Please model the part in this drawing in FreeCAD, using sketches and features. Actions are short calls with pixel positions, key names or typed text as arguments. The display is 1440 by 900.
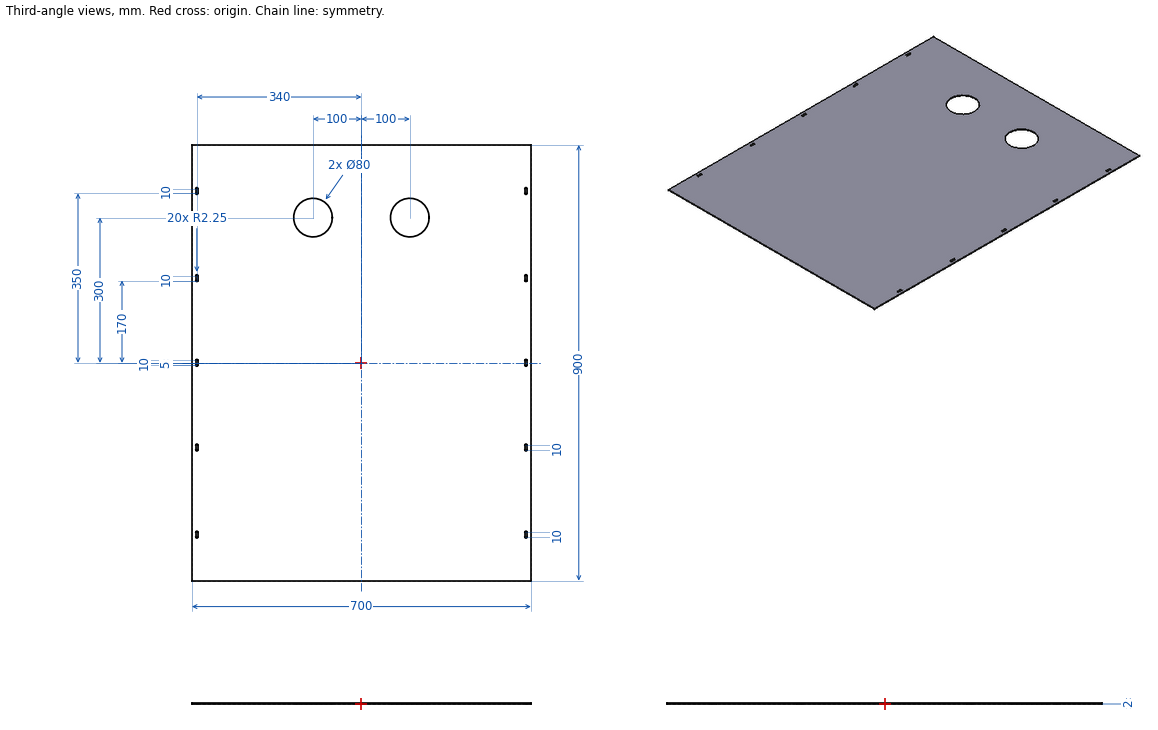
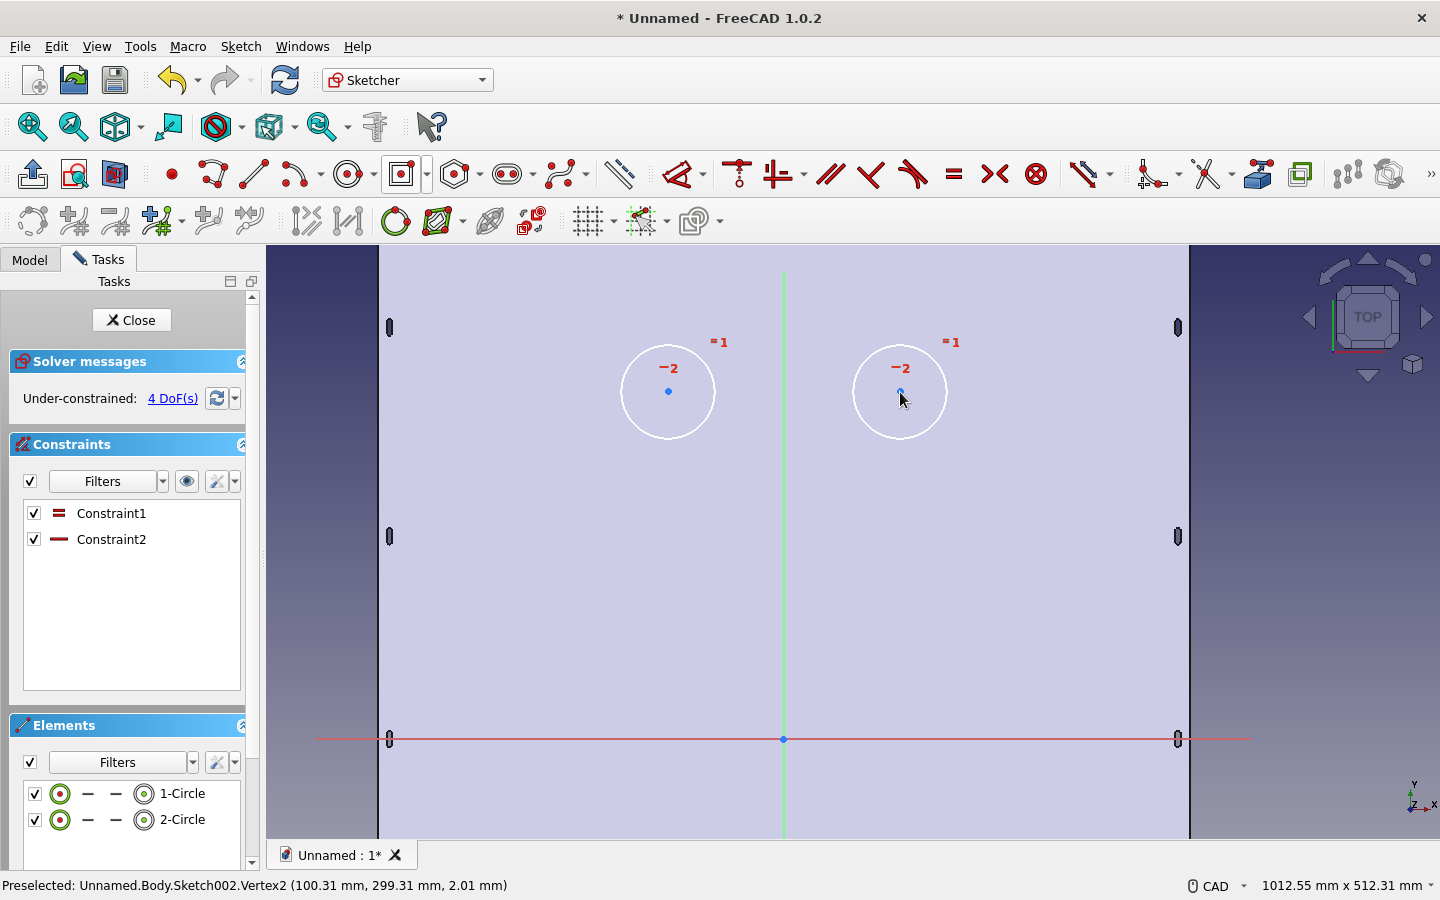
key(d)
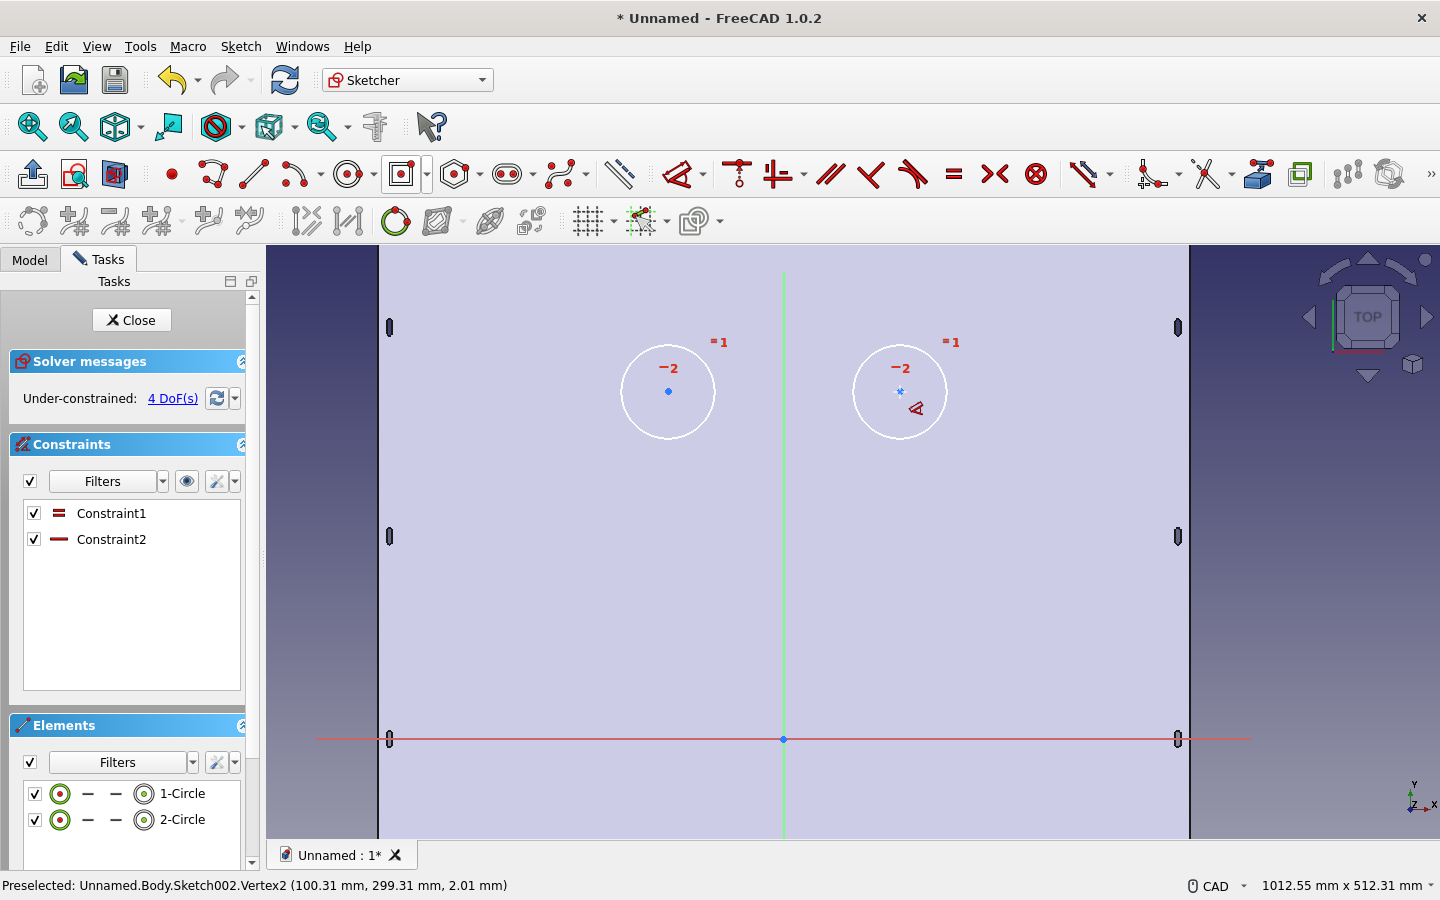
click(701, 359)
click(724, 336)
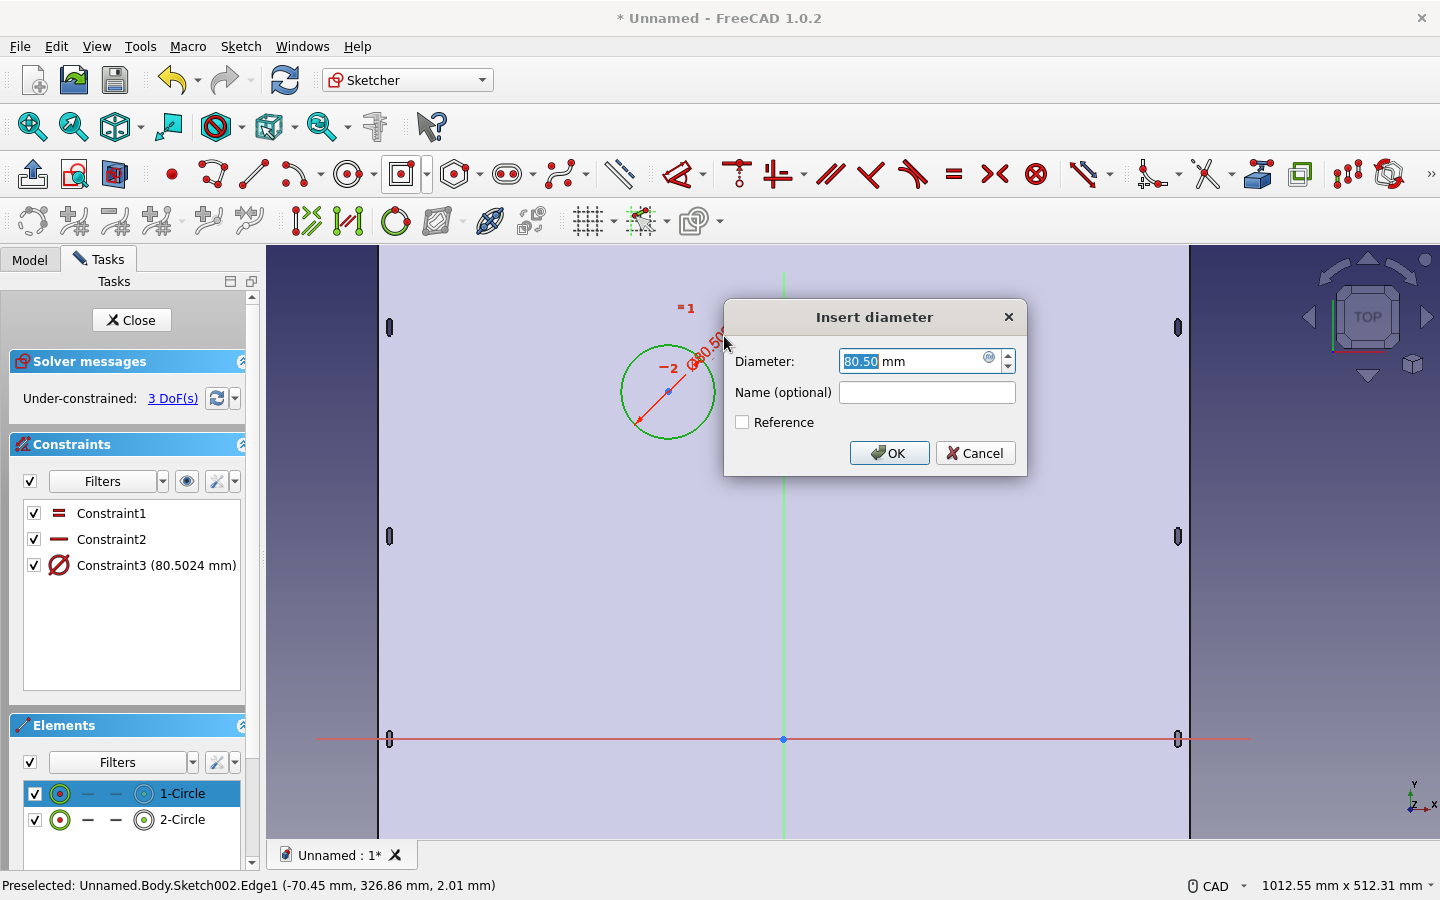
text(80)
key(Return)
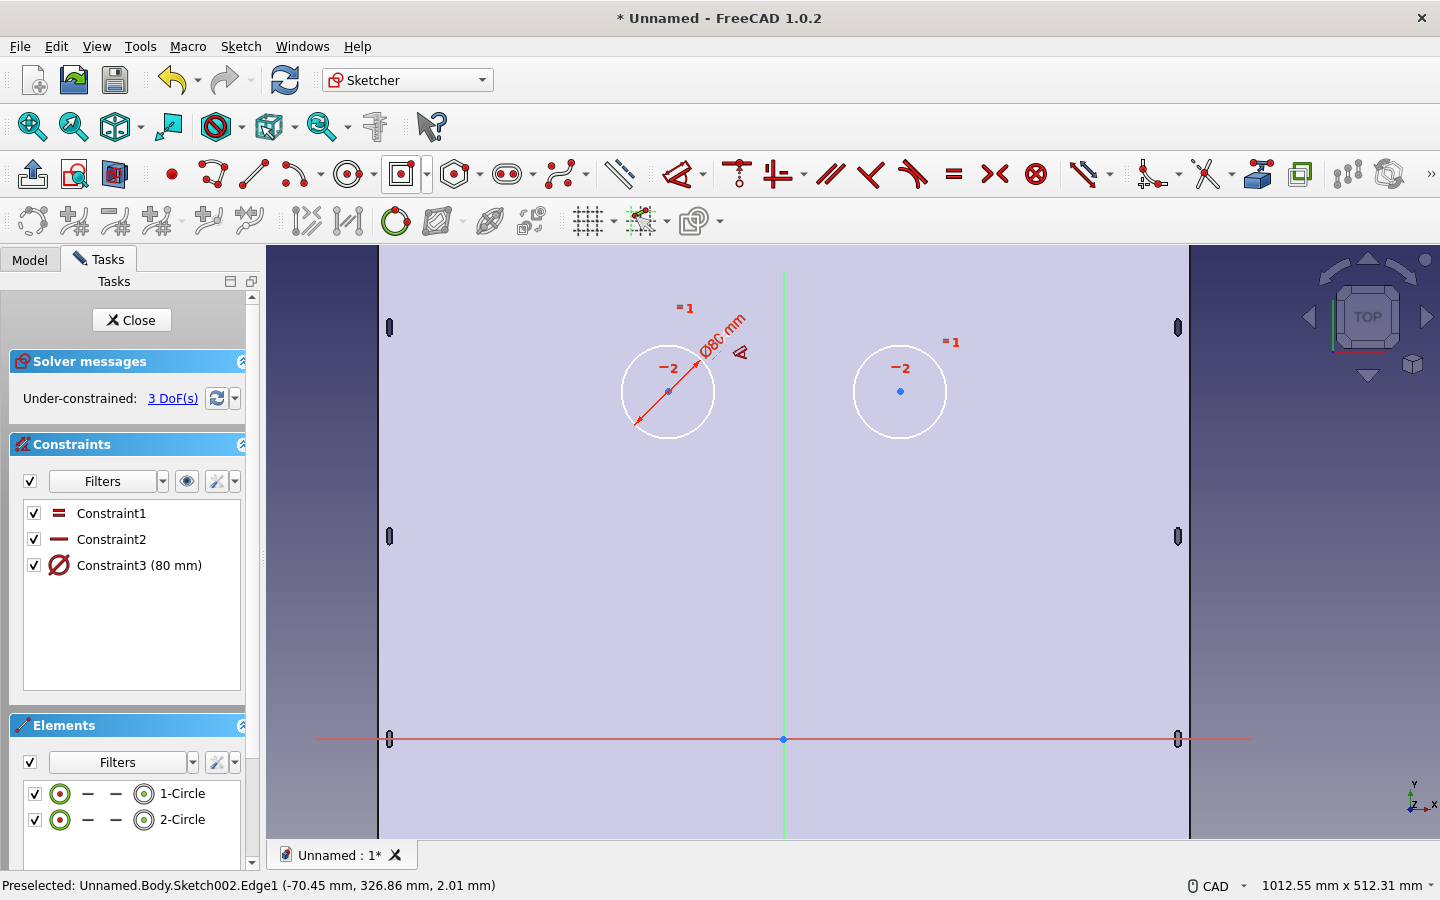
click(668, 392)
click(726, 773)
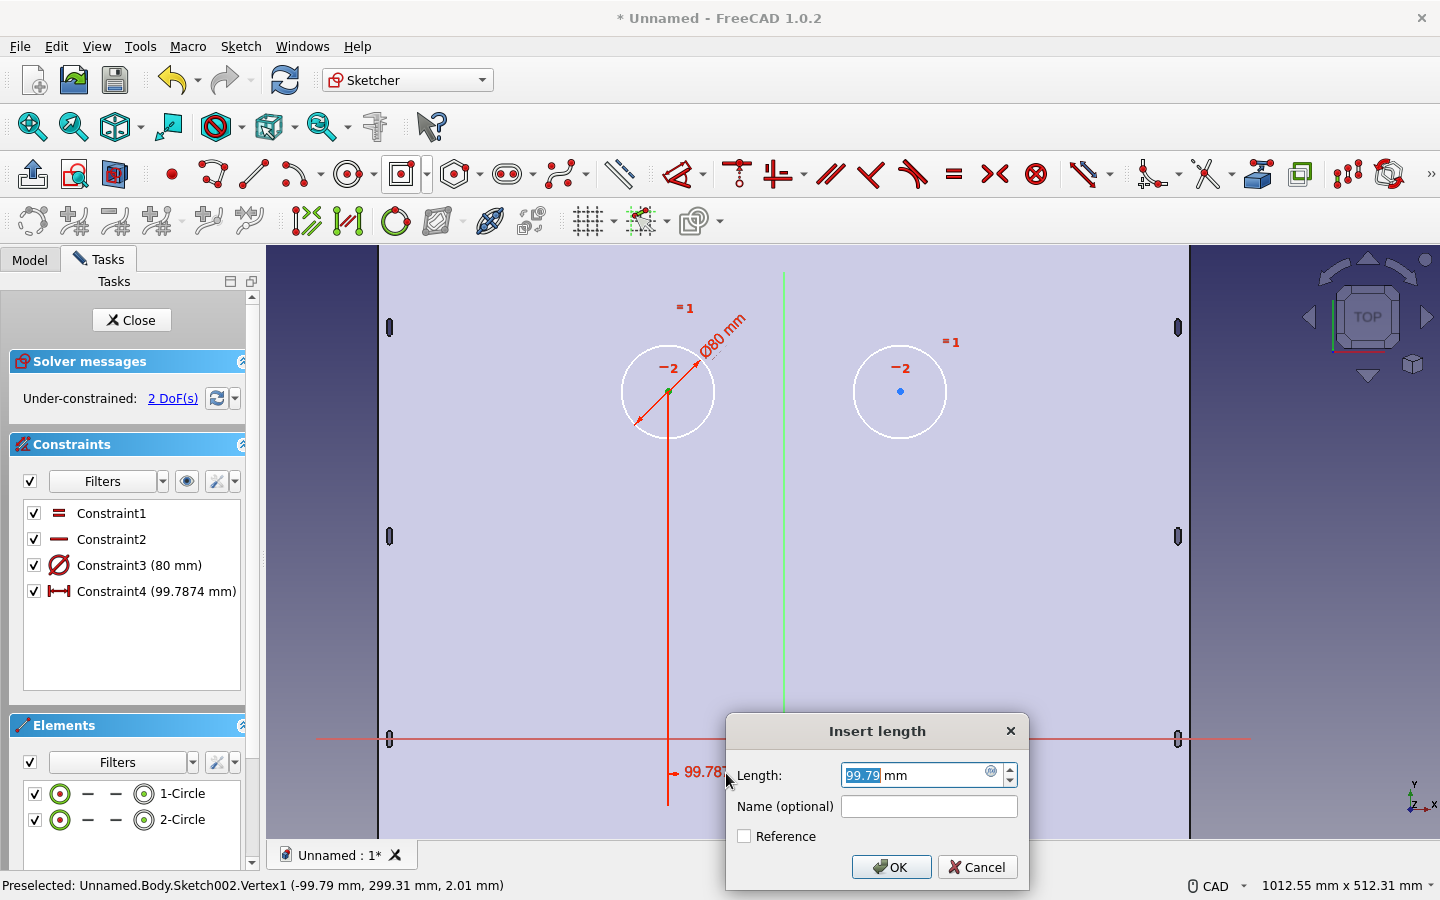
text(100)
key(Return)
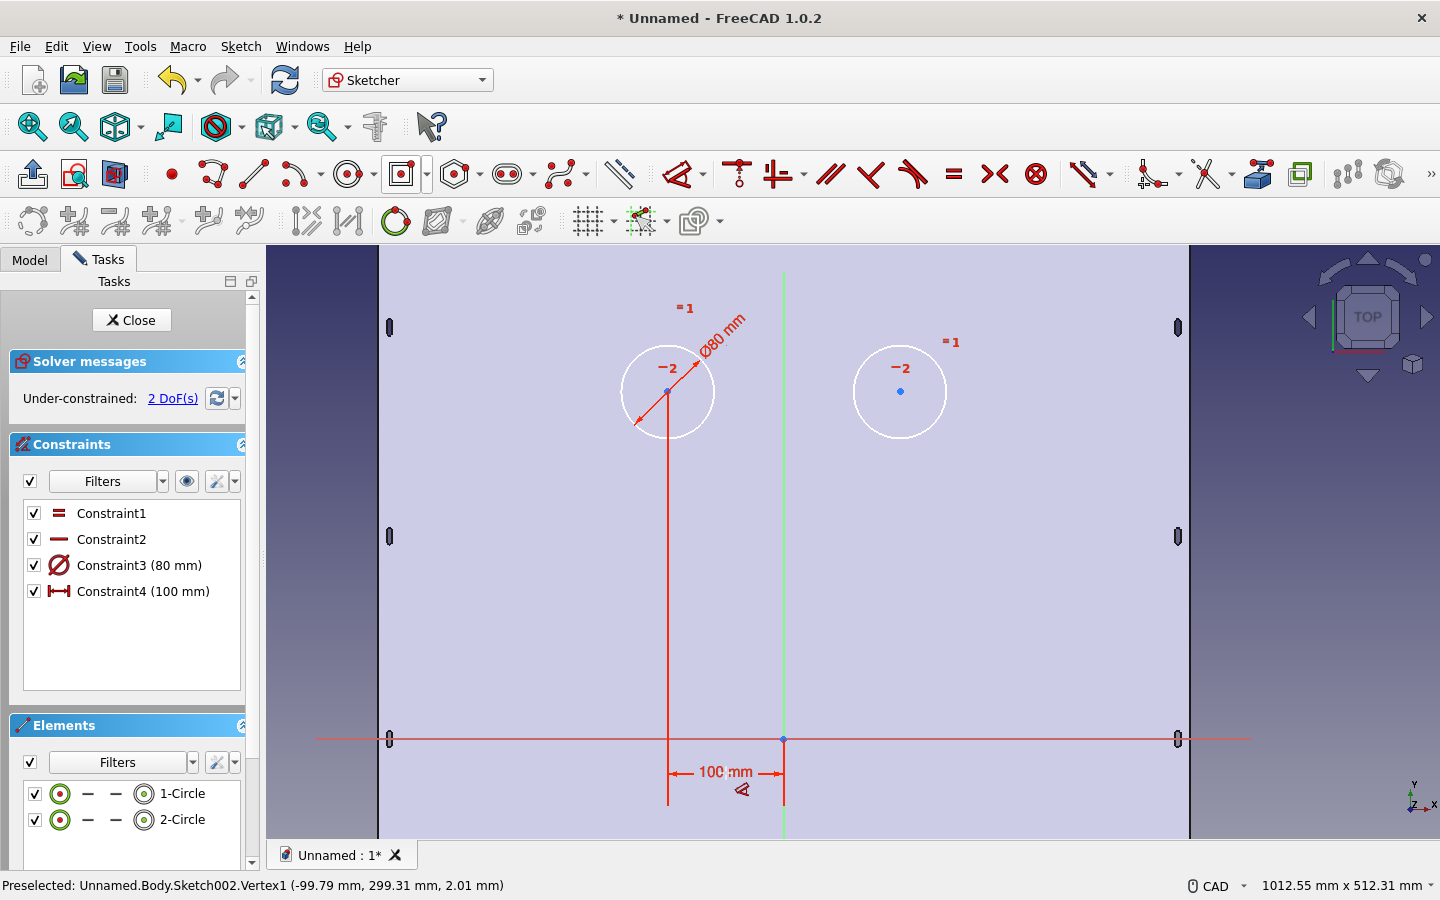
click(668, 392)
click(634, 566)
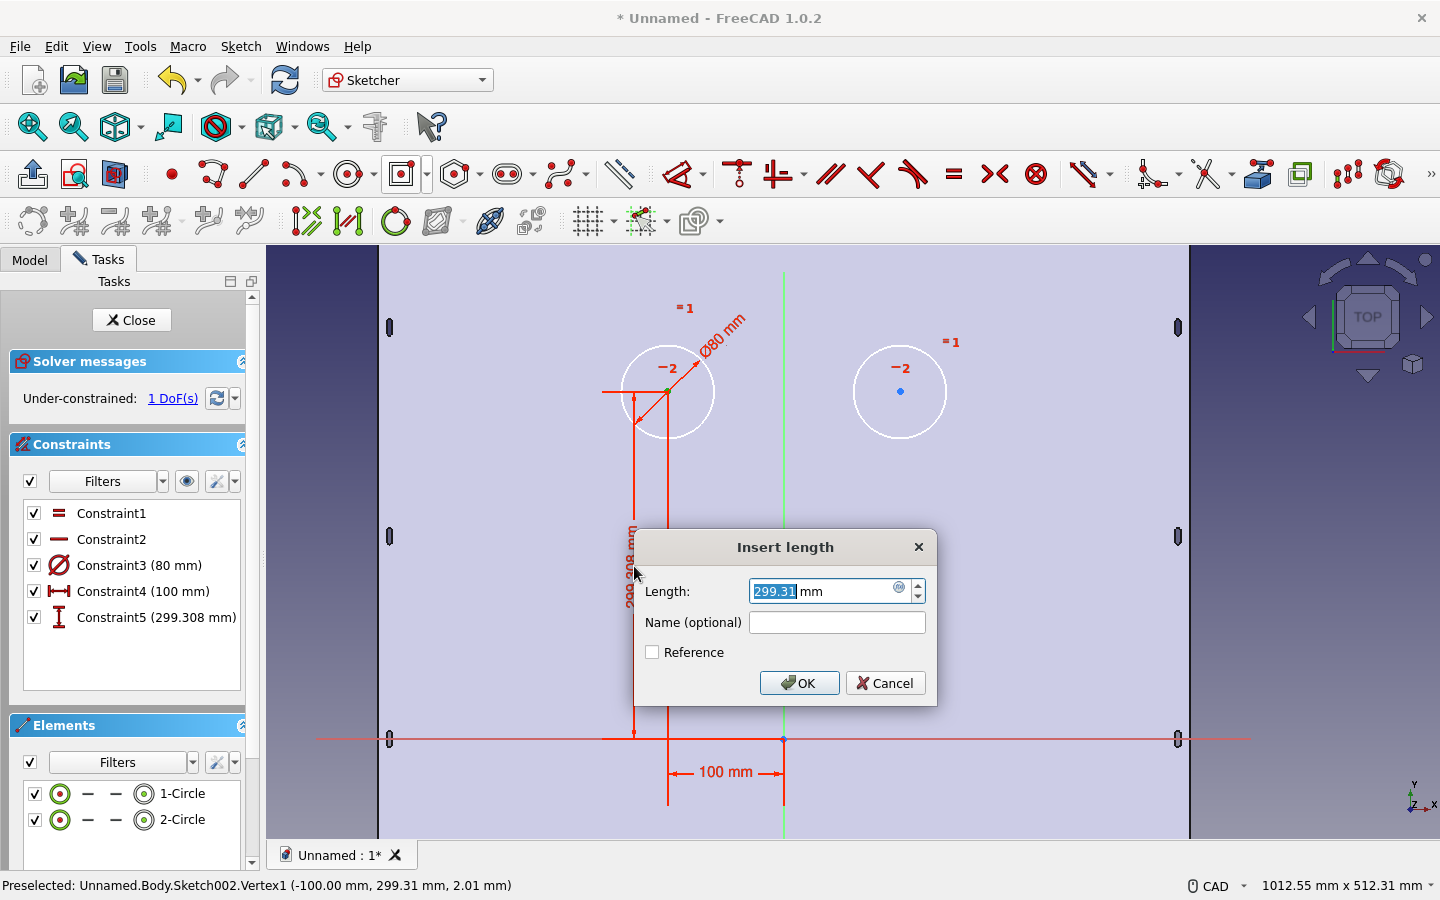
text(300)
key(Return)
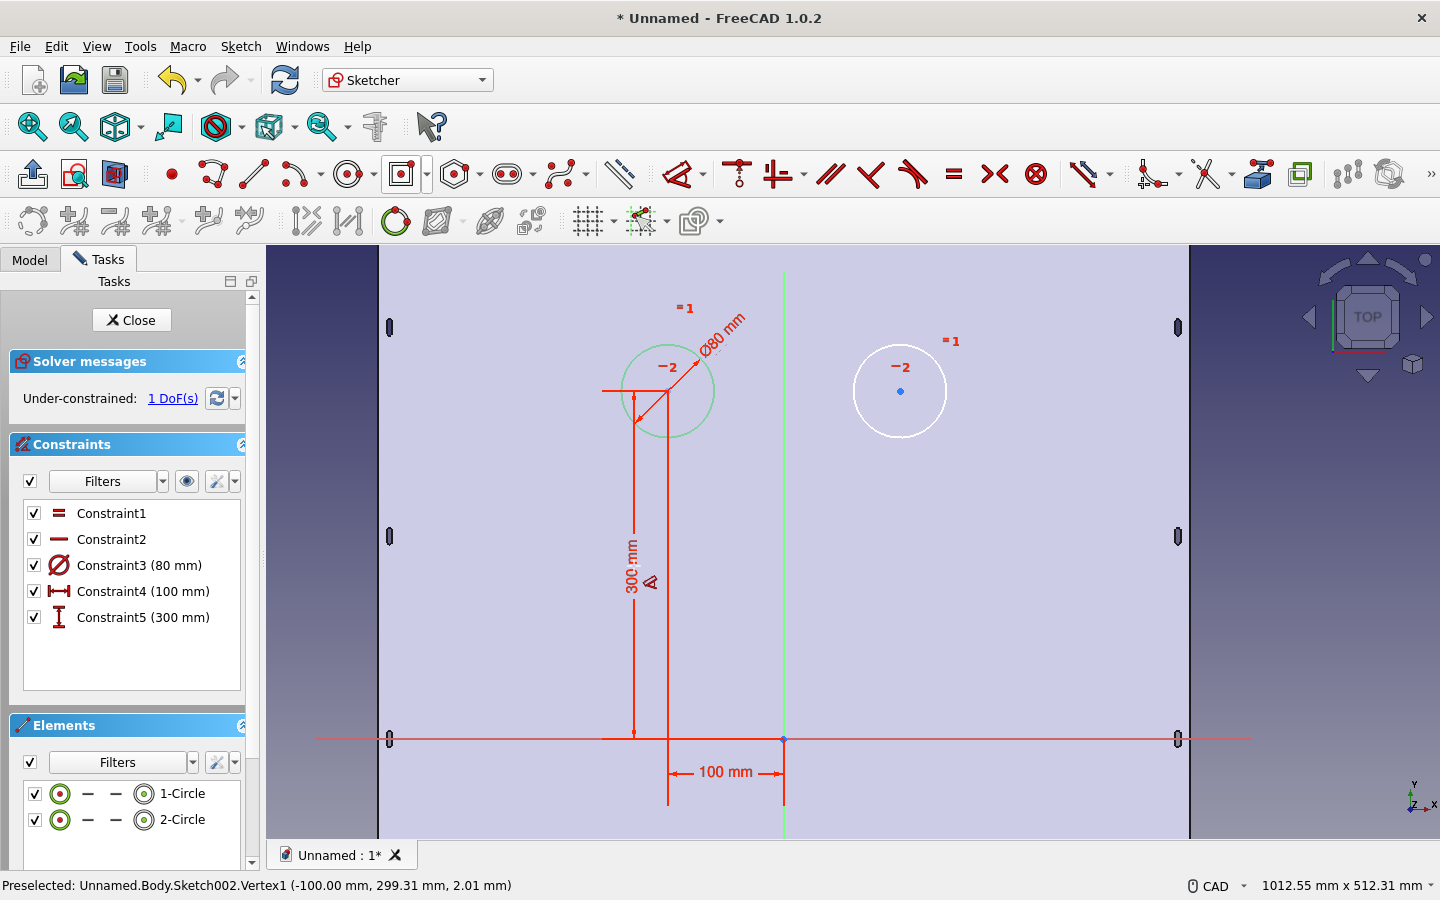
click(900, 391)
click(842, 773)